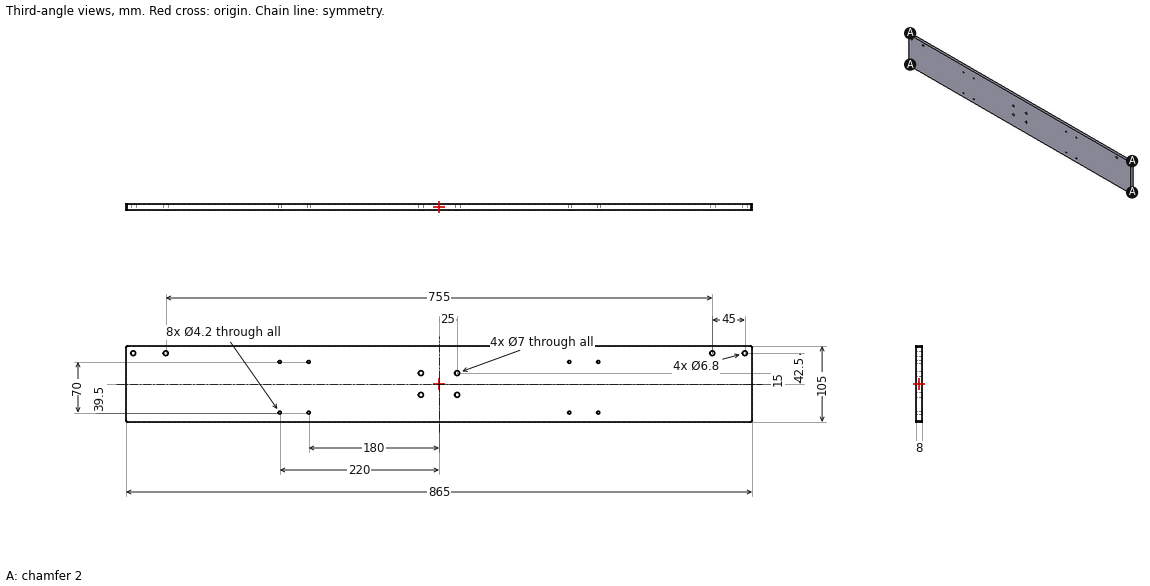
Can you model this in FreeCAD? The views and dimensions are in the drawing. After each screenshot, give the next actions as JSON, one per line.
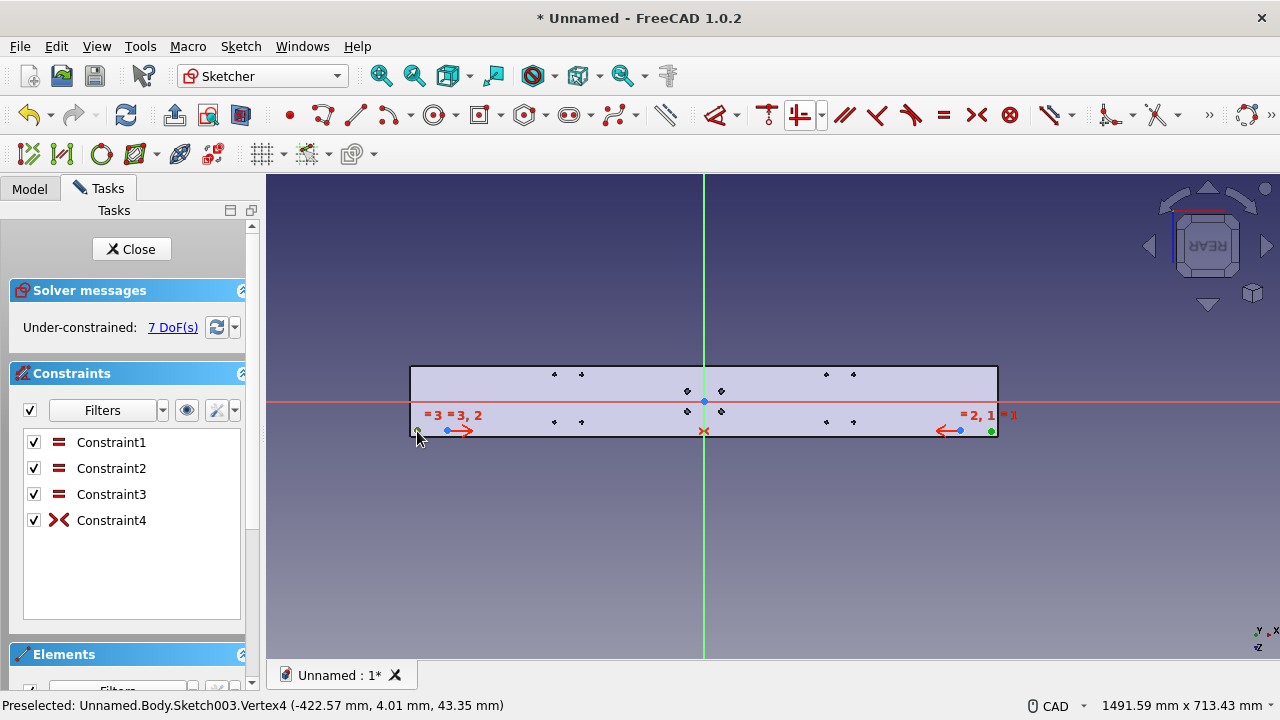
{"action": "left_click", "coordinate": [704, 600]}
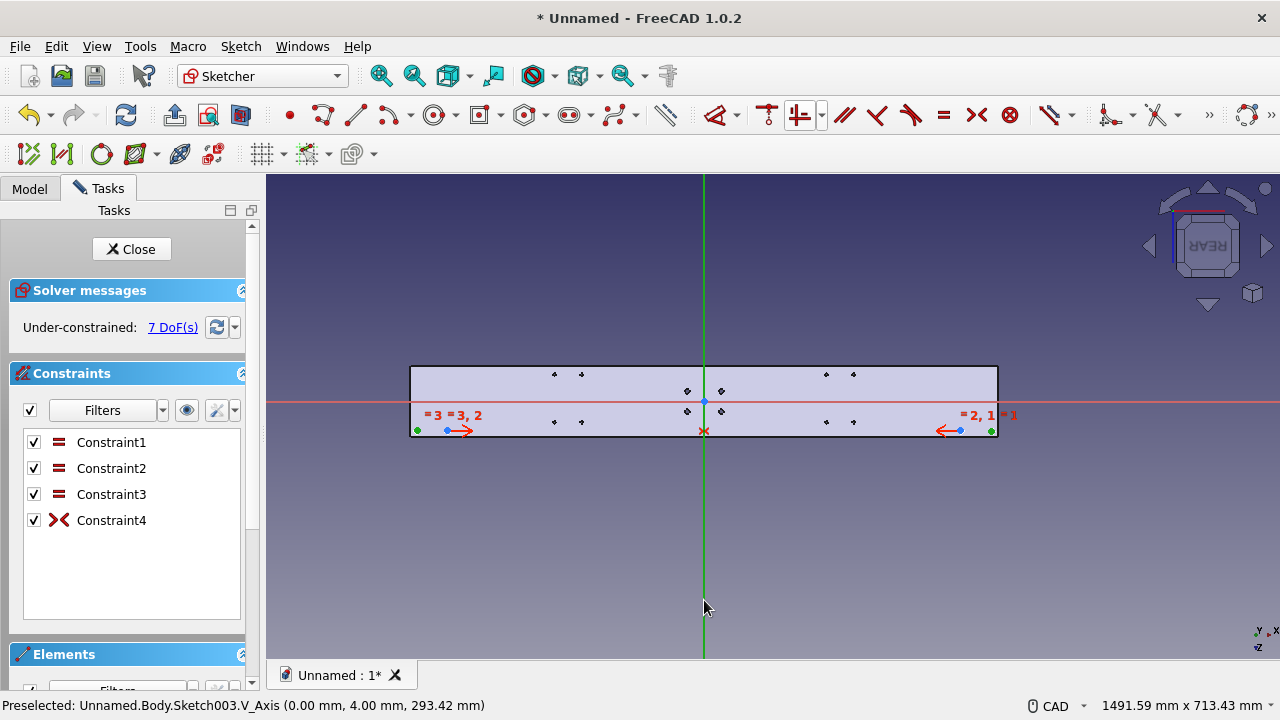
{"action": "key", "text": "s"}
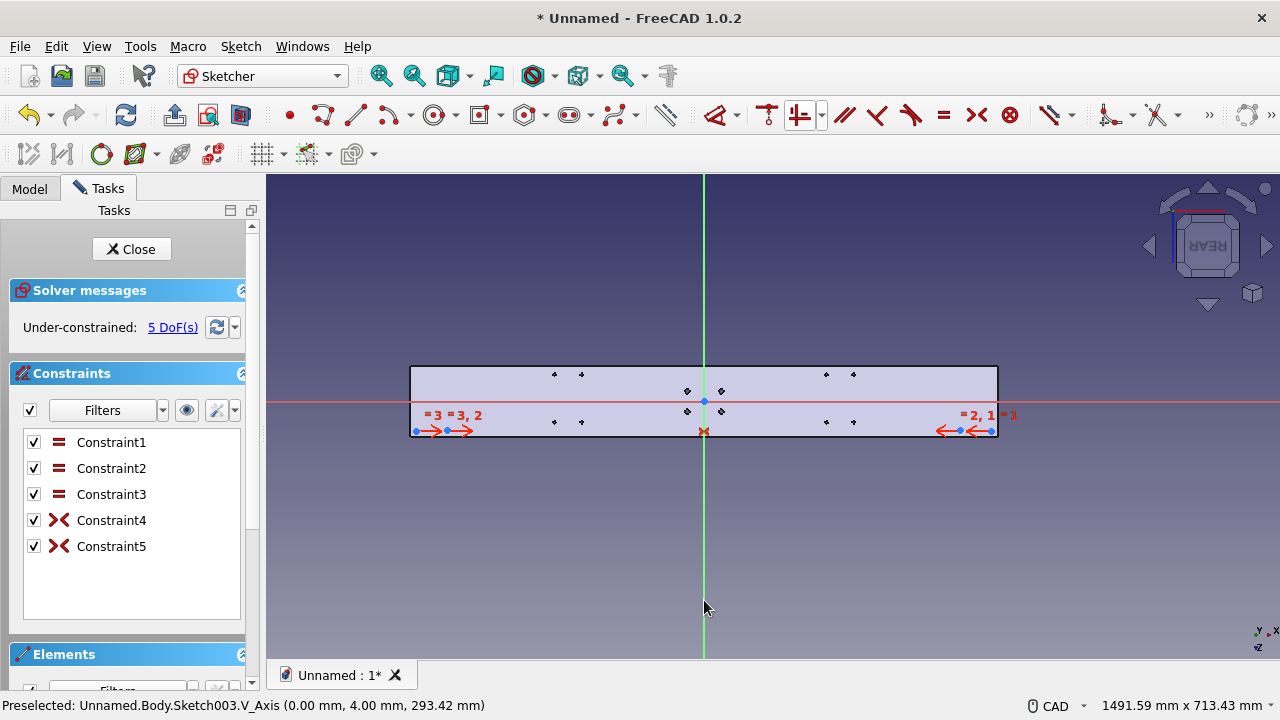
{"action": "key", "text": "d"}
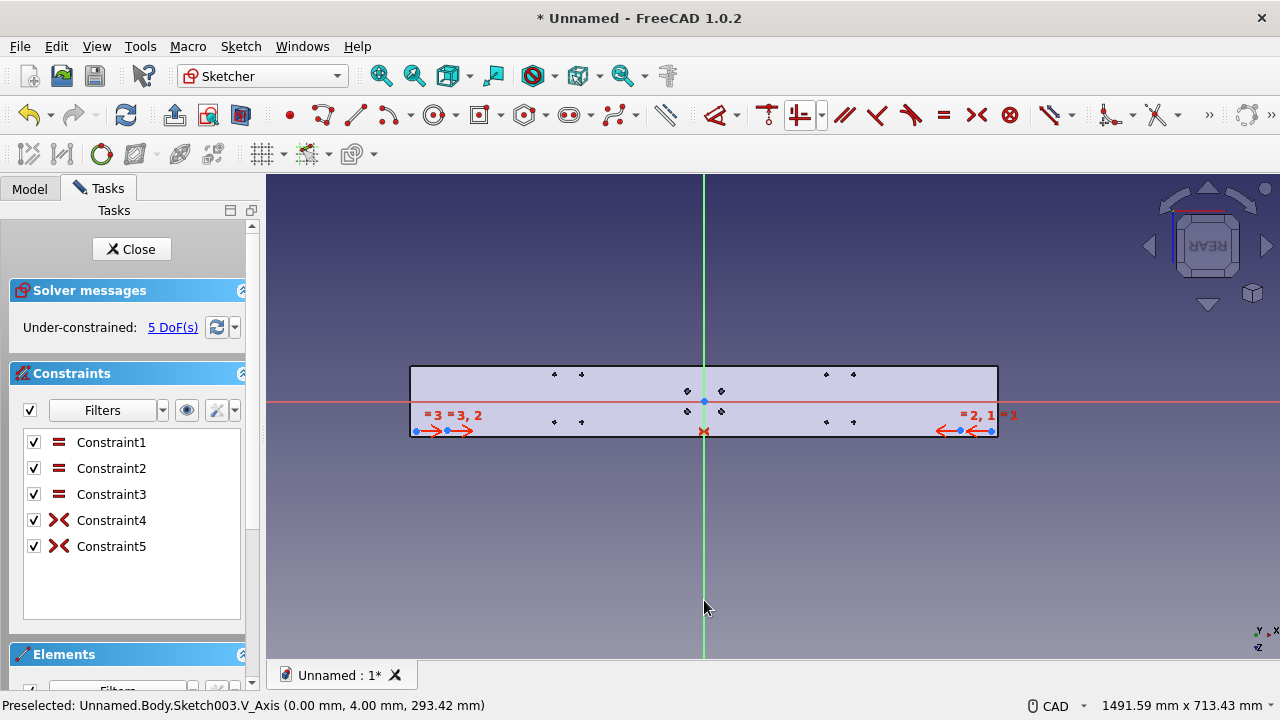
{"action": "scroll", "coordinate": [992, 429], "scroll_direction": "up", "scroll_amount": 11}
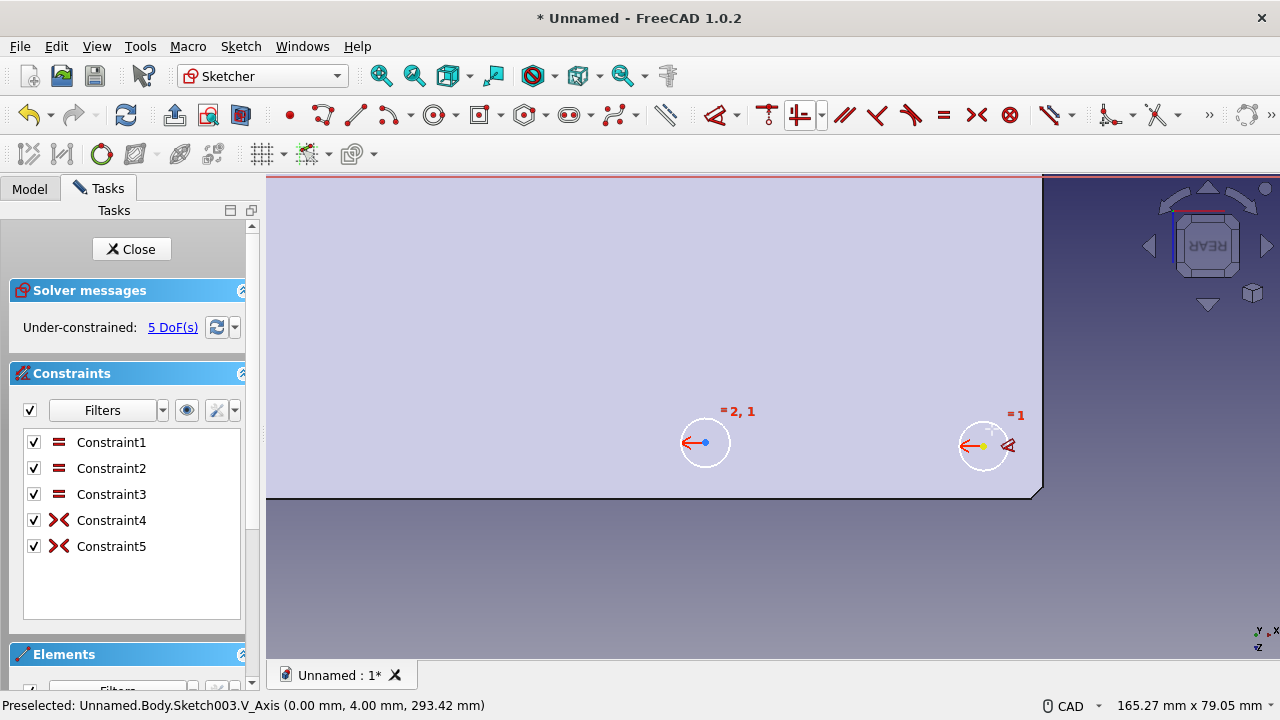
{"action": "left_click", "coordinate": [984, 422]}
{"action": "left_click", "coordinate": [984, 390]}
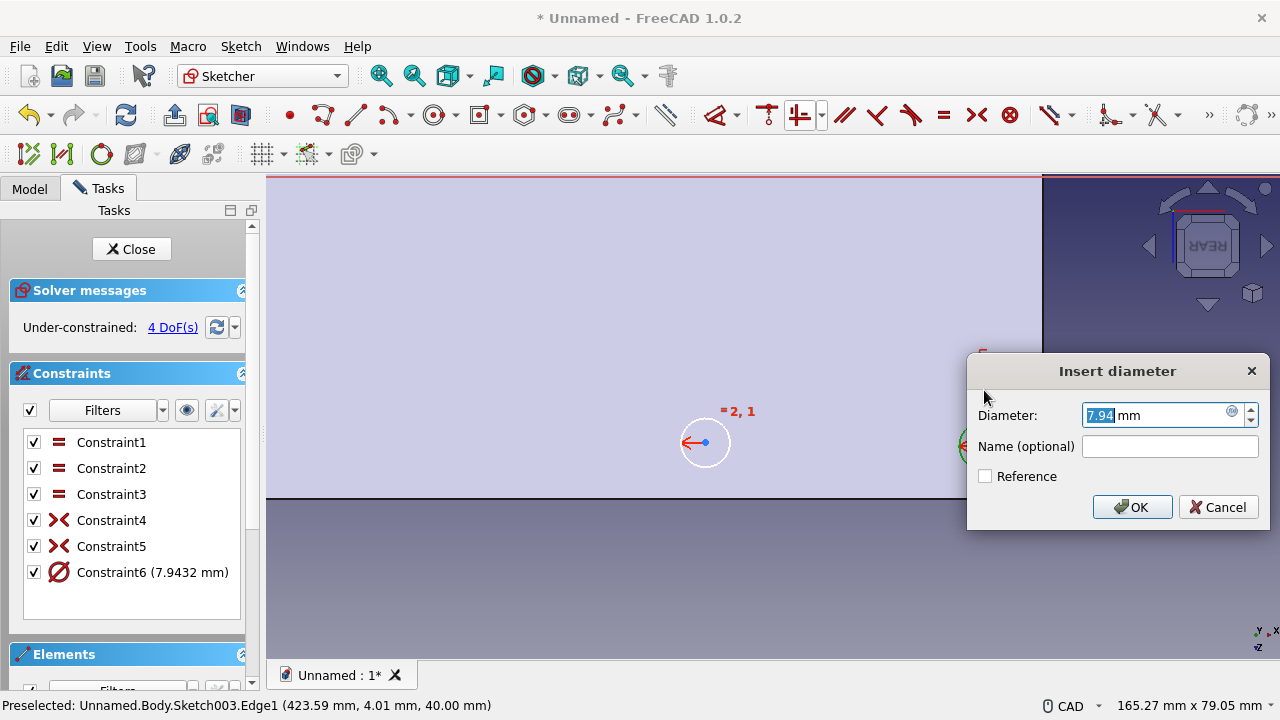
{"action": "type", "text": "6.8"}
{"action": "key", "text": "Return"}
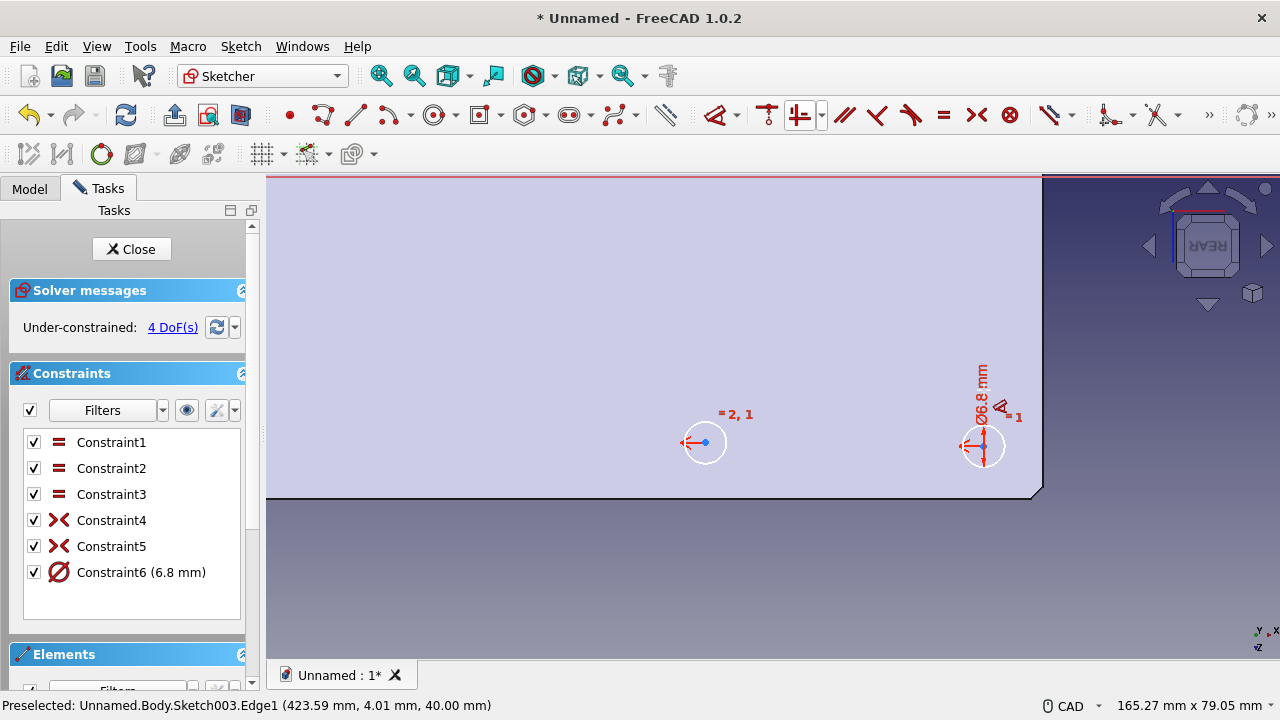
{"action": "scroll", "coordinate": [993, 429], "scroll_direction": "down", "scroll_amount": 11}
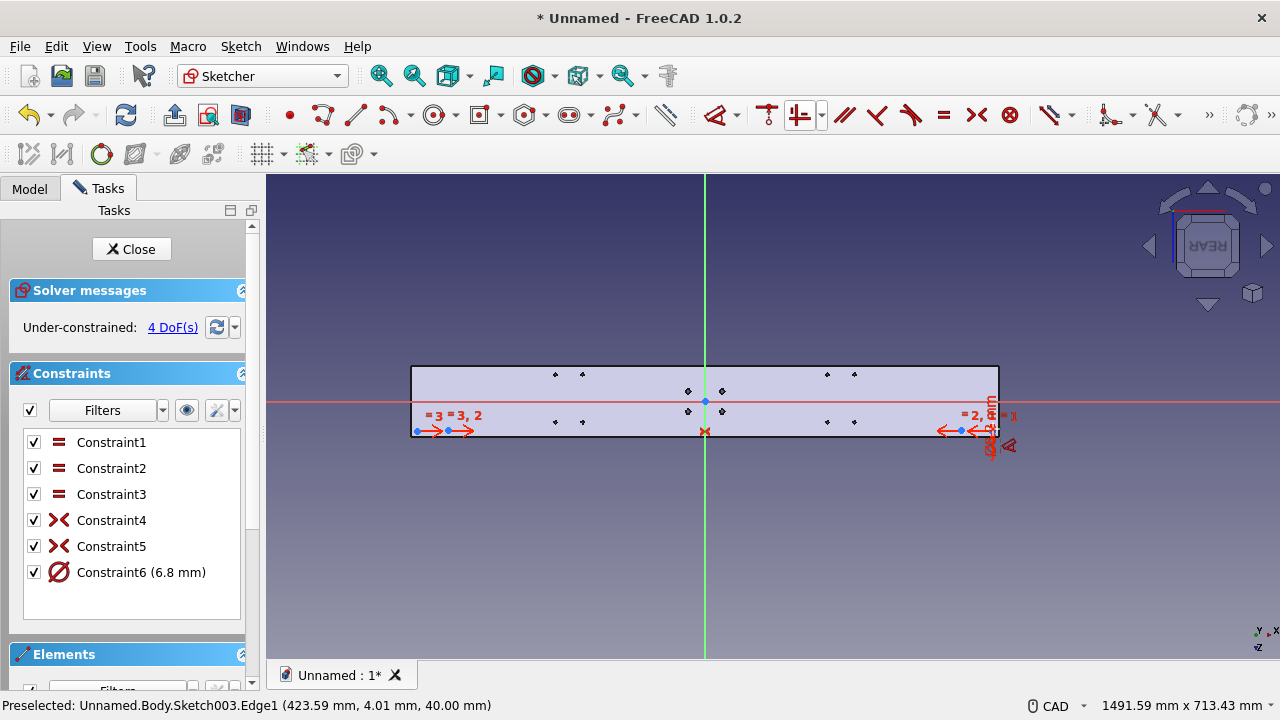
{"action": "scroll", "coordinate": [993, 431], "scroll_direction": "up", "scroll_amount": 2}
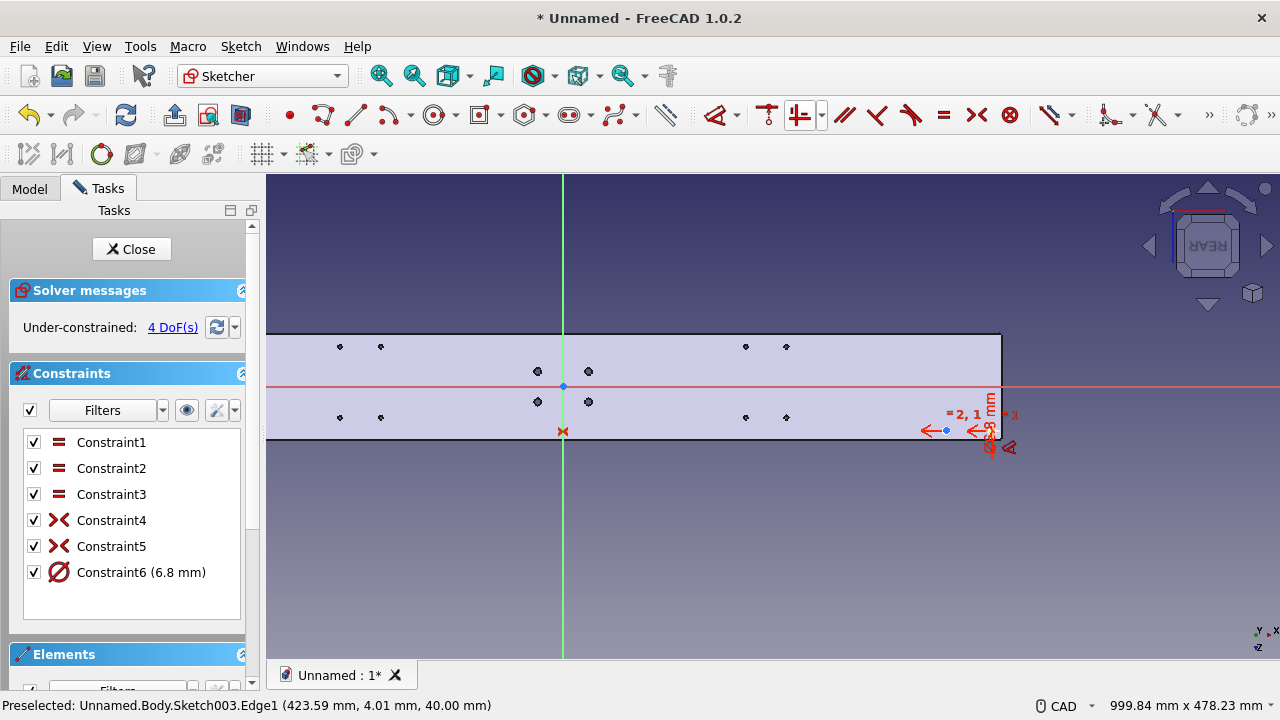
{"action": "left_click", "coordinate": [992, 431]}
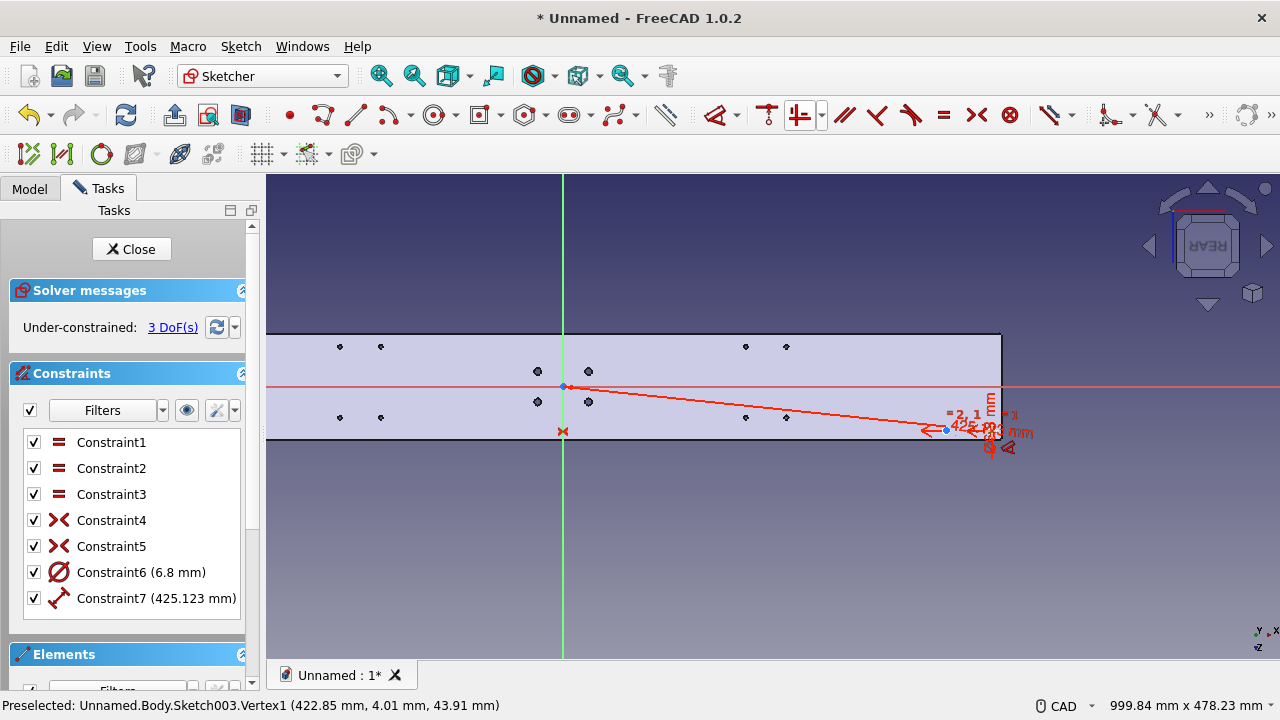
{"action": "left_click", "coordinate": [946, 431]}
{"action": "left_click", "coordinate": [969, 465]}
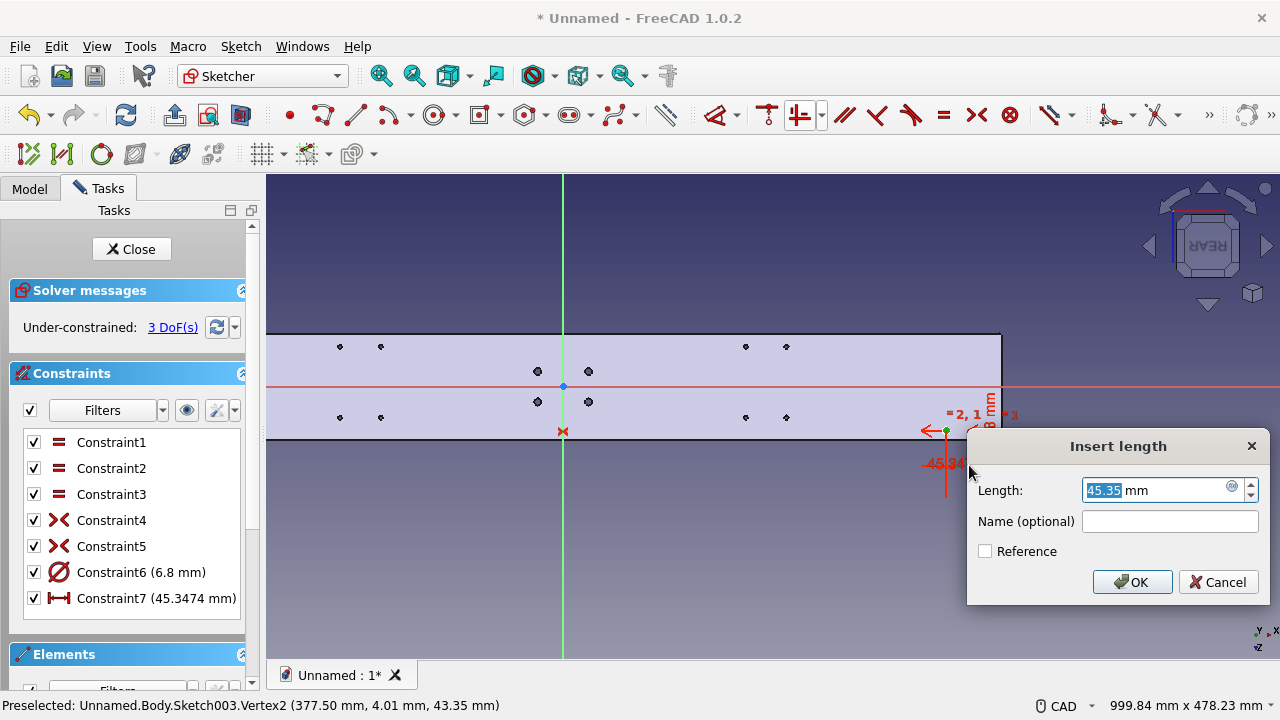
{"action": "type", "text": "45"}
{"action": "key", "text": "Return"}